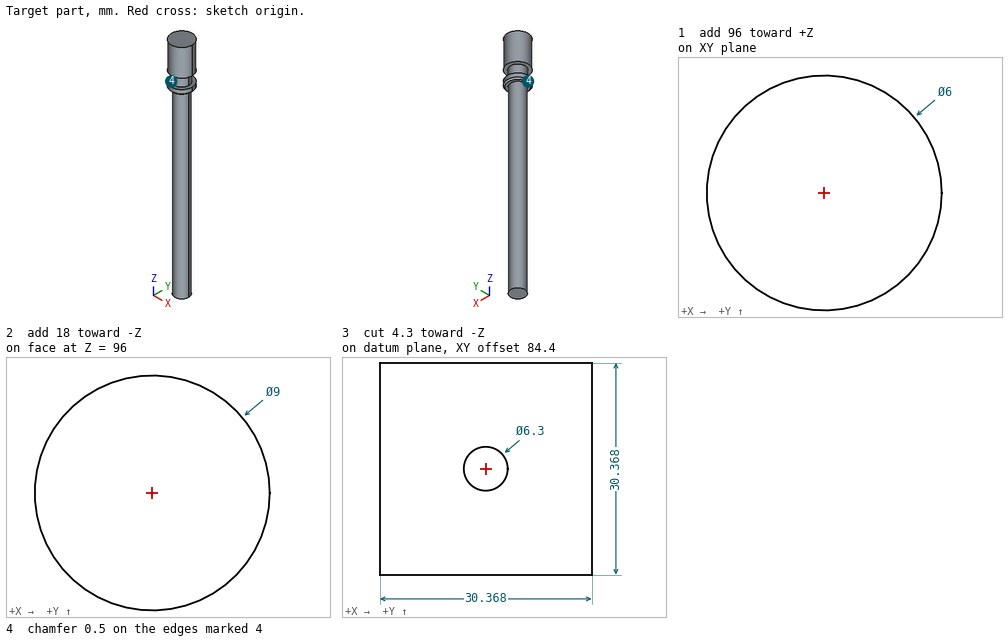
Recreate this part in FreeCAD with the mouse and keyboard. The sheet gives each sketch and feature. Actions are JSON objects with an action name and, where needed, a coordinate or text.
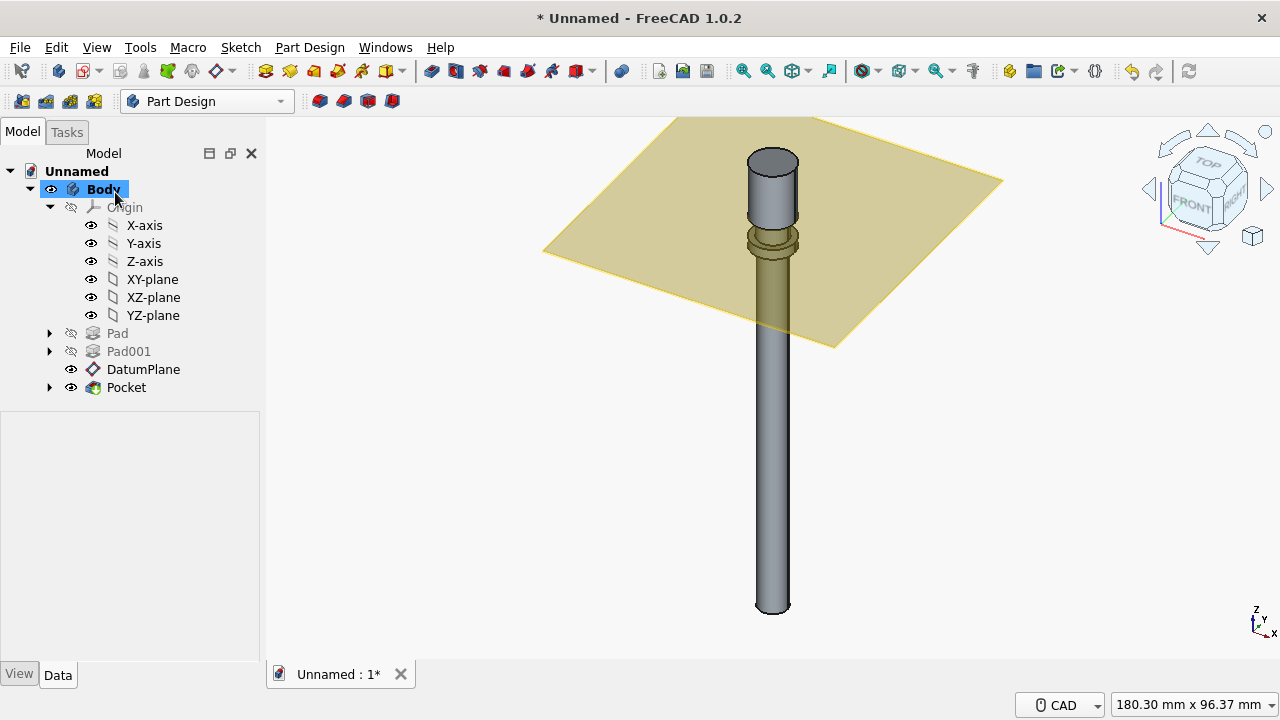
{"action": "left_click", "coordinate": [116, 369]}
{"action": "key", "text": "space"}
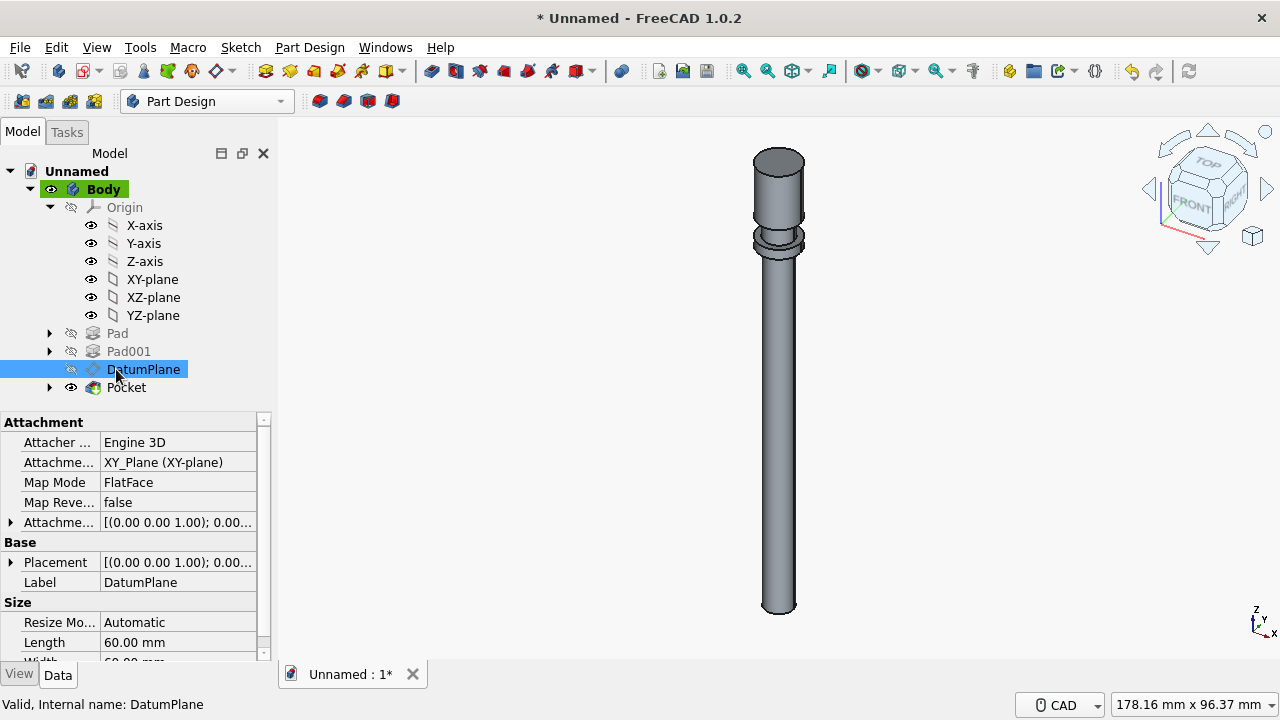
{"action": "left_click", "coordinate": [760, 254]}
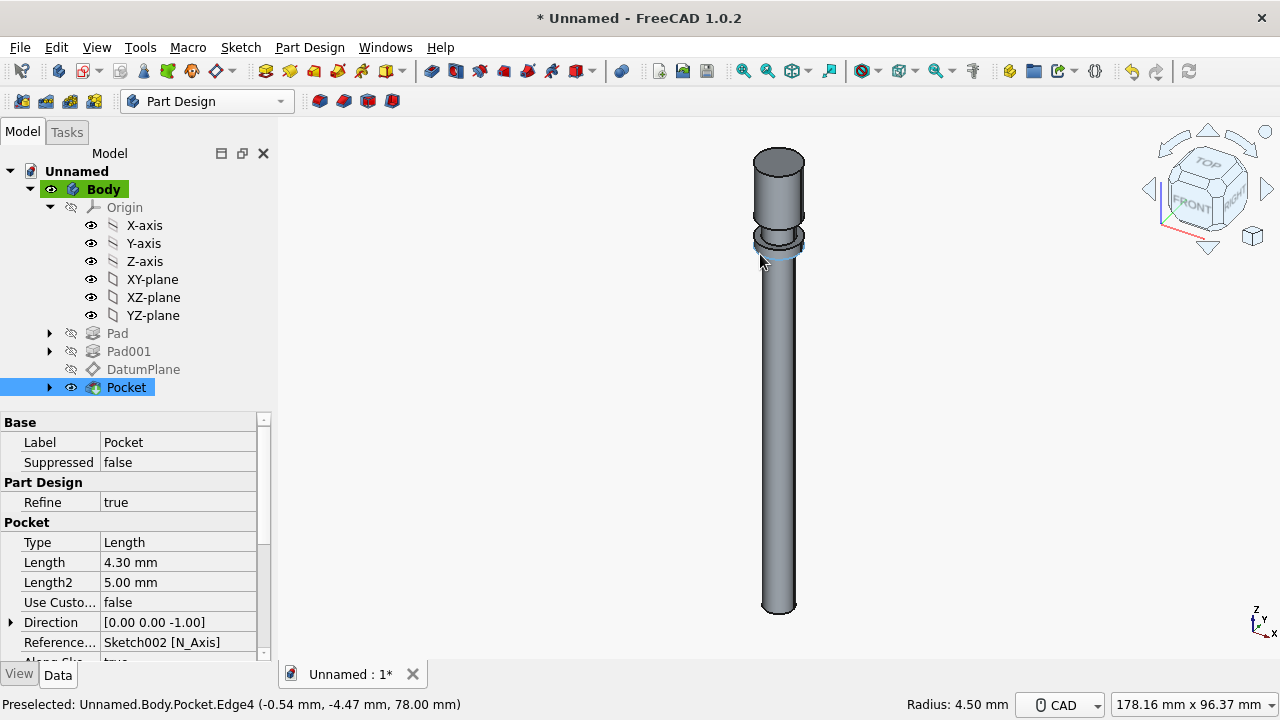
{"action": "left_click", "coordinate": [344, 102]}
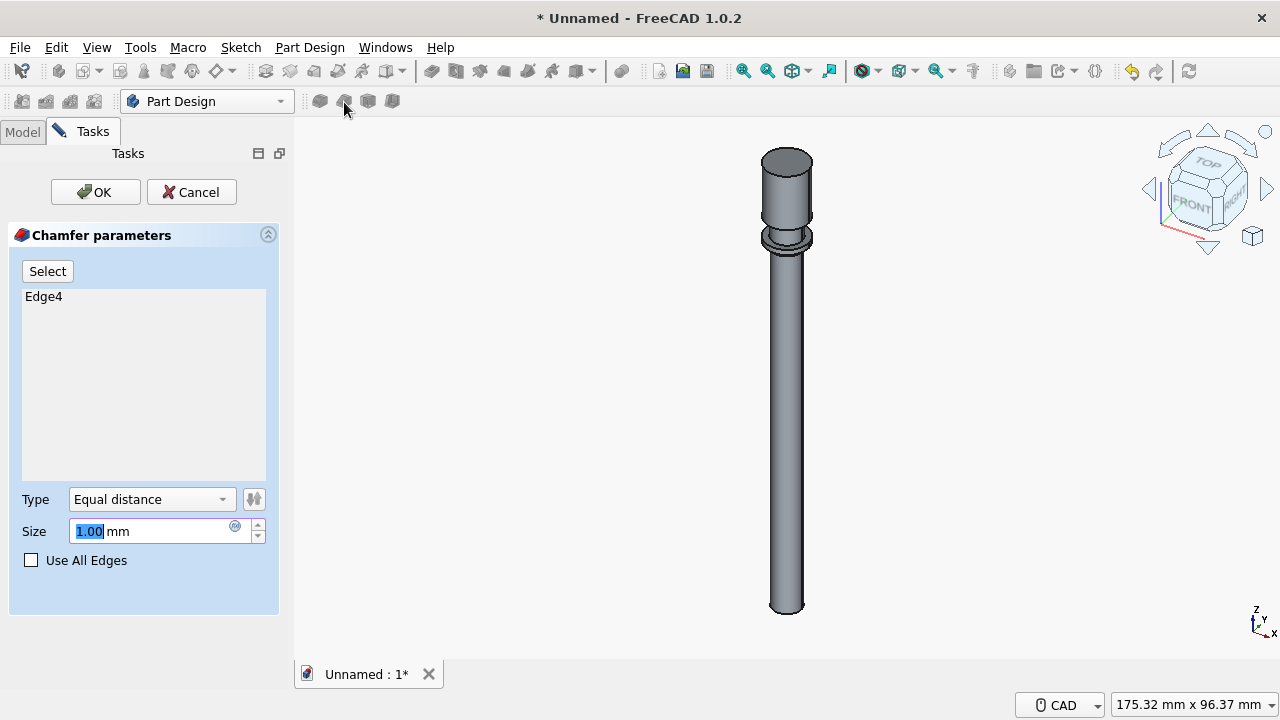
{"action": "type", "text": "0.5"}
{"action": "key", "text": "Tab"}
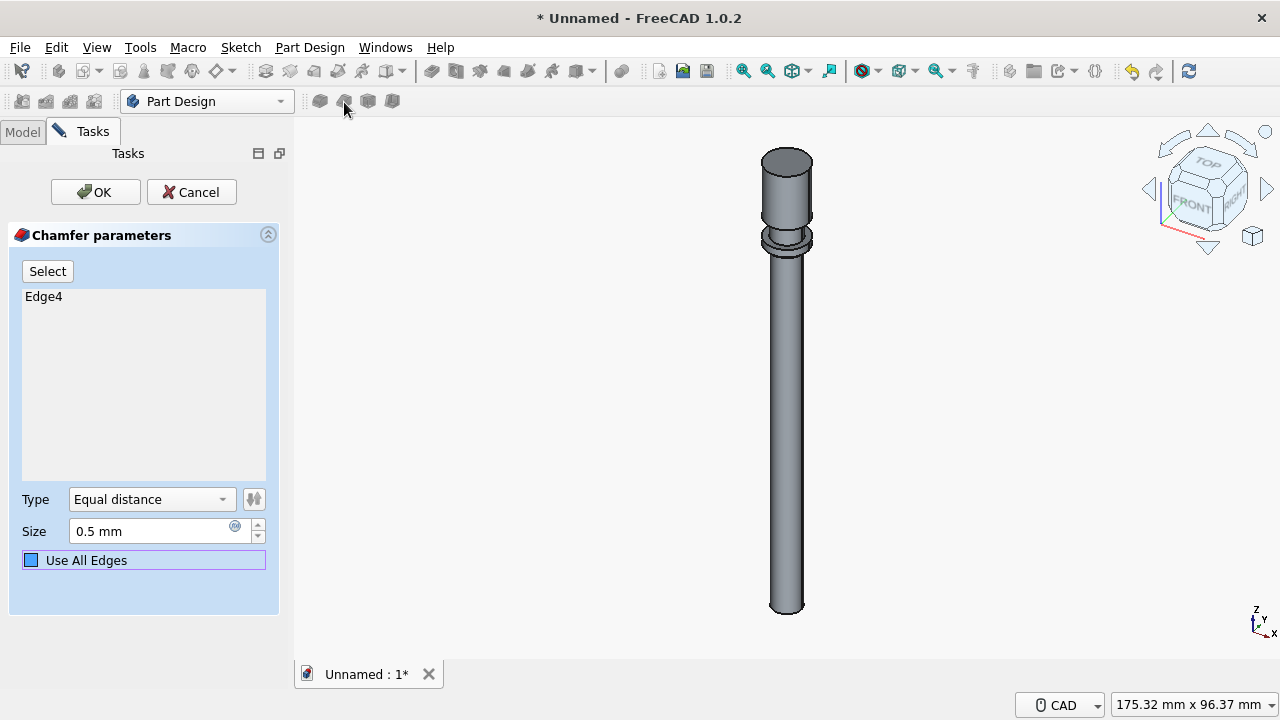
{"action": "left_click", "coordinate": [96, 192]}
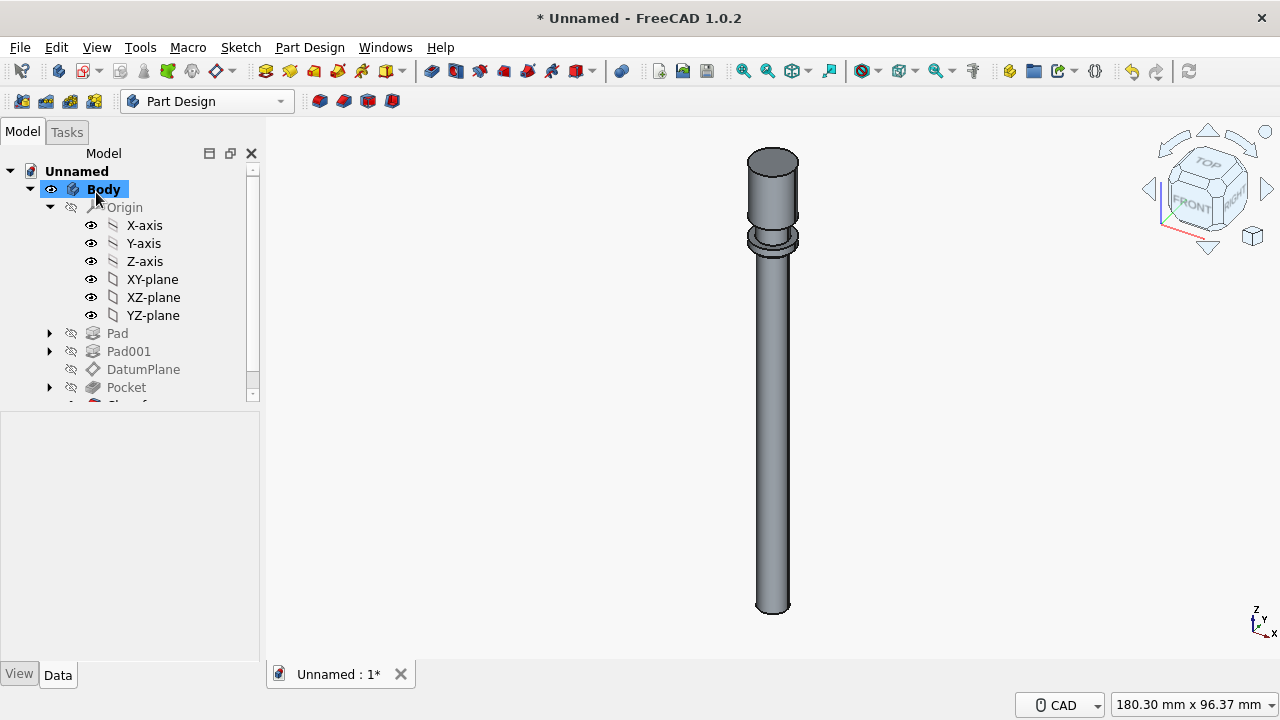
{"action": "key", "text": "0"}